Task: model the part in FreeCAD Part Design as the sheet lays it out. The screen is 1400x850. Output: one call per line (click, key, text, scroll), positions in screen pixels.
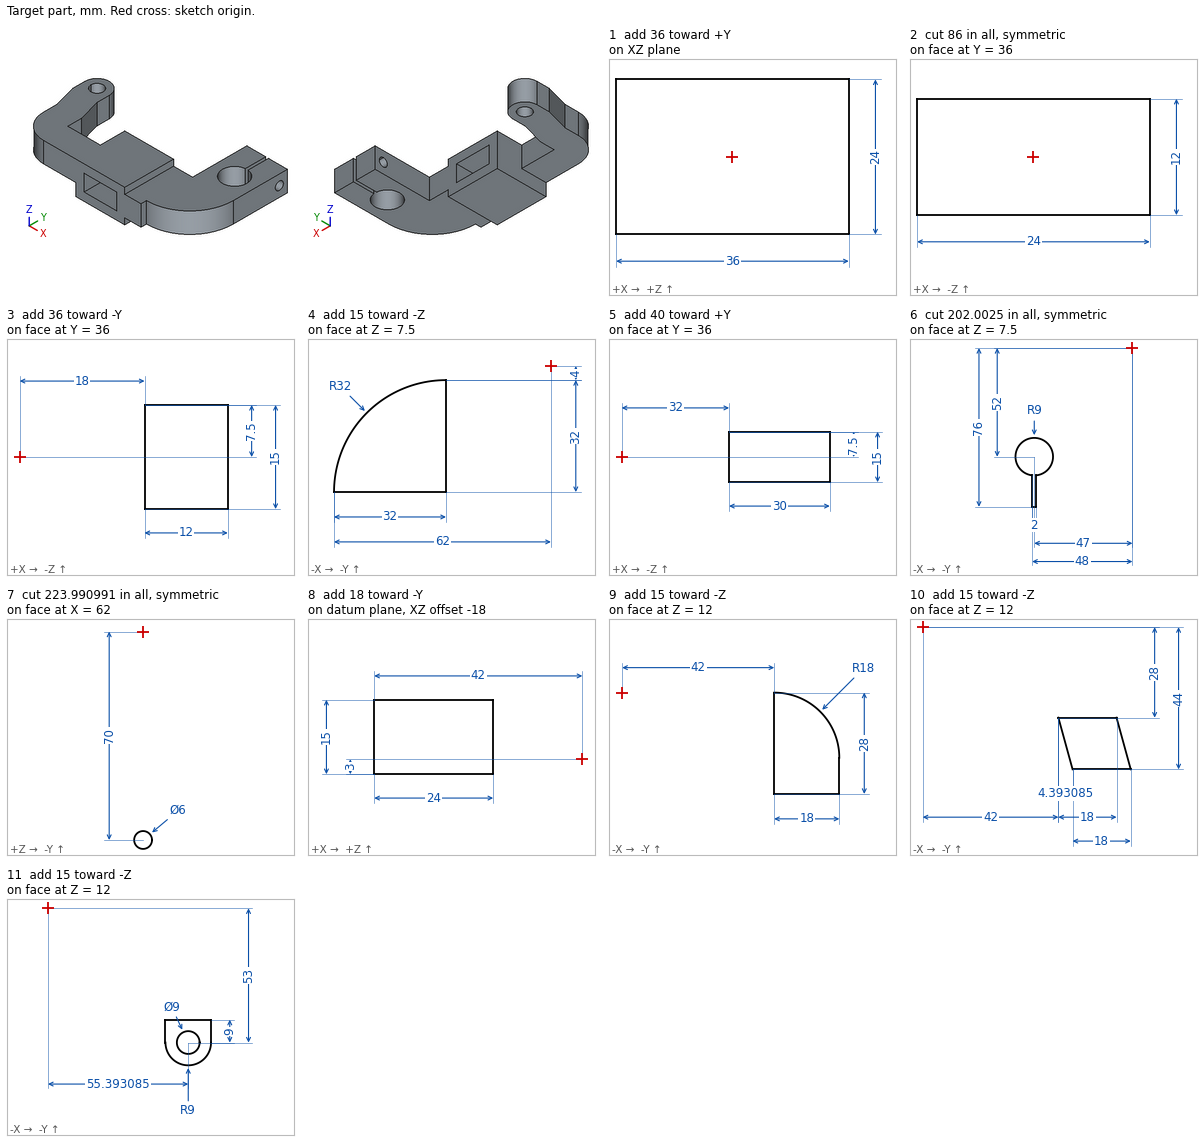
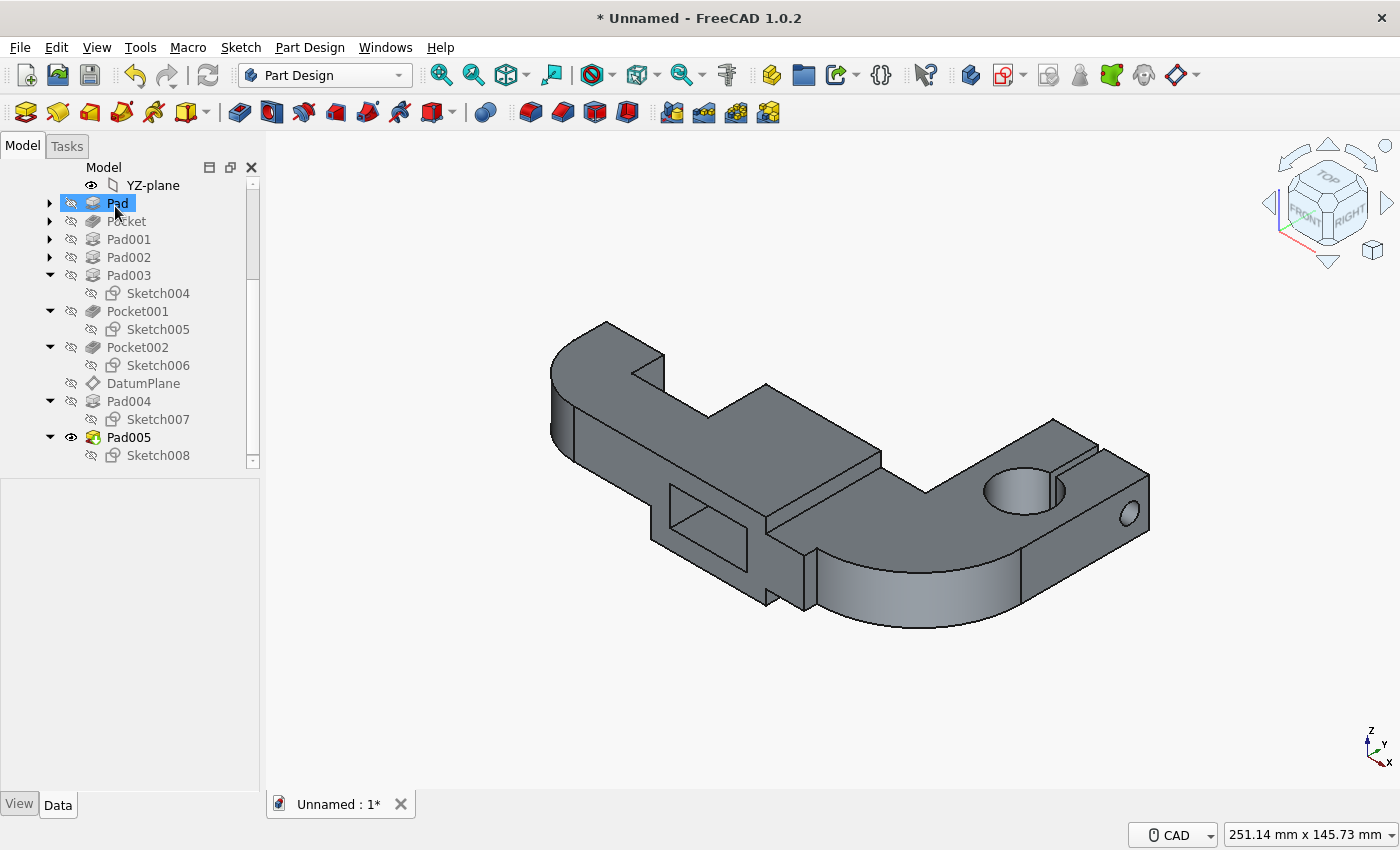
click(770, 452)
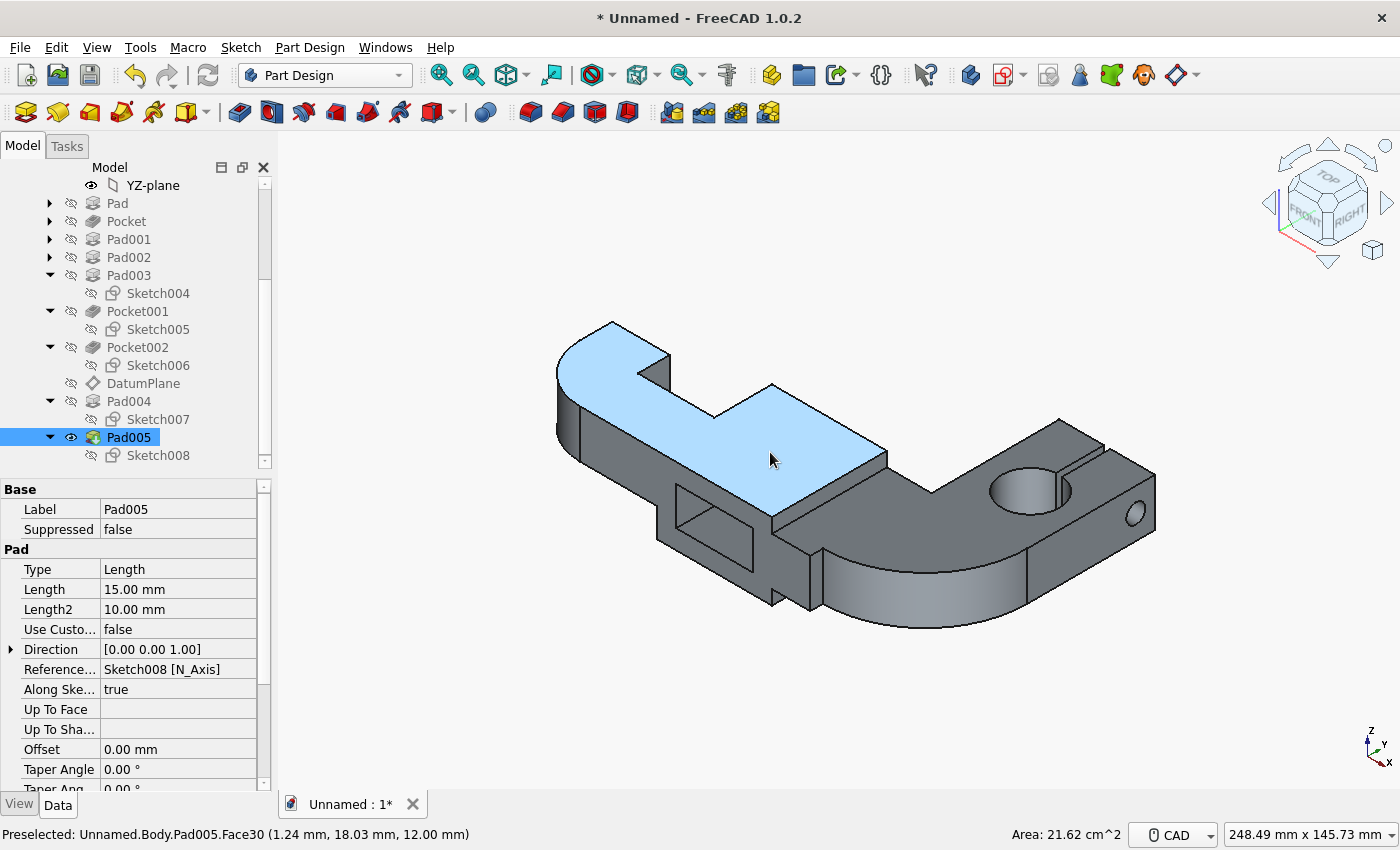
click(1004, 76)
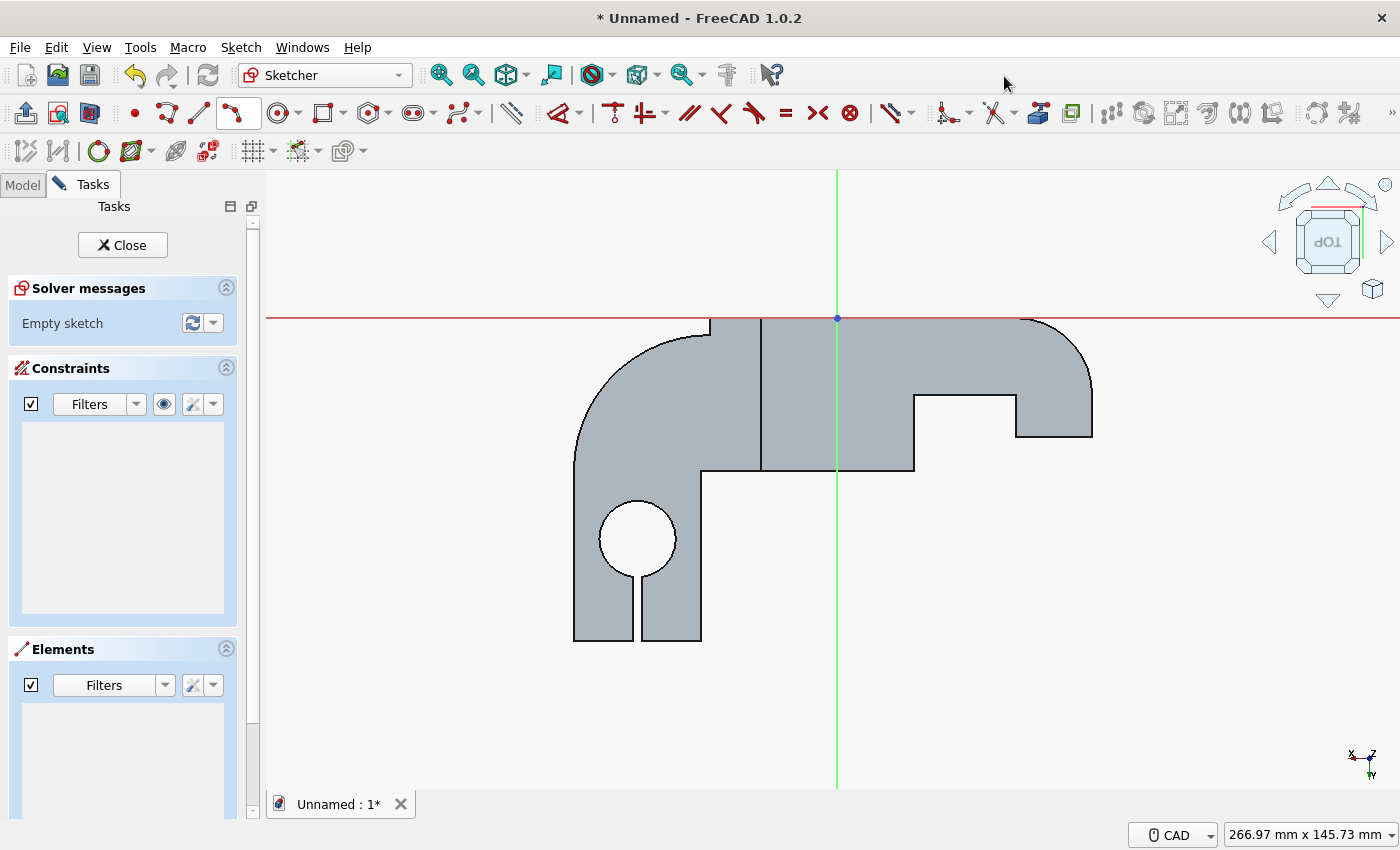
scroll(1122, 469, up, 9)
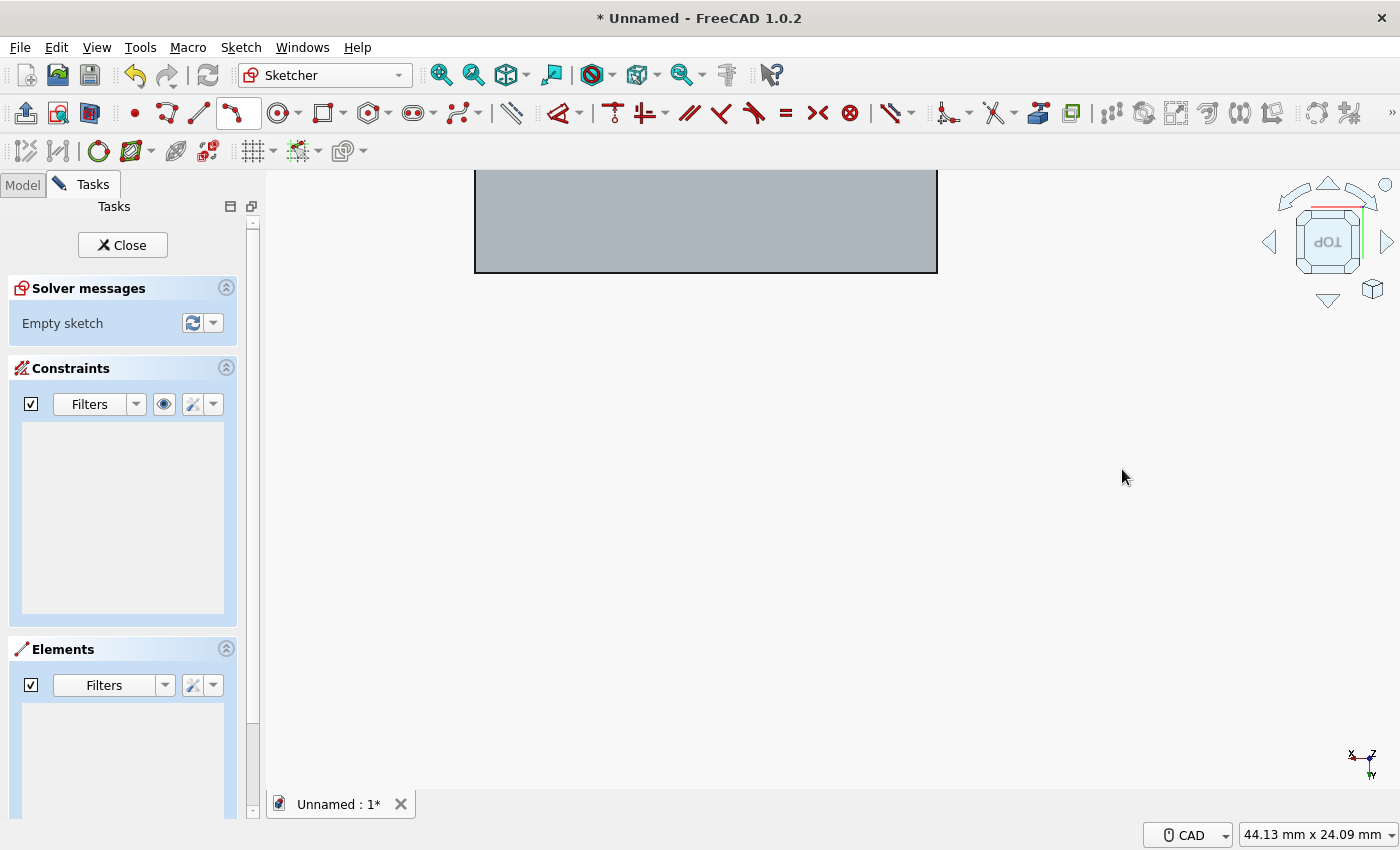
key(g)
key(m)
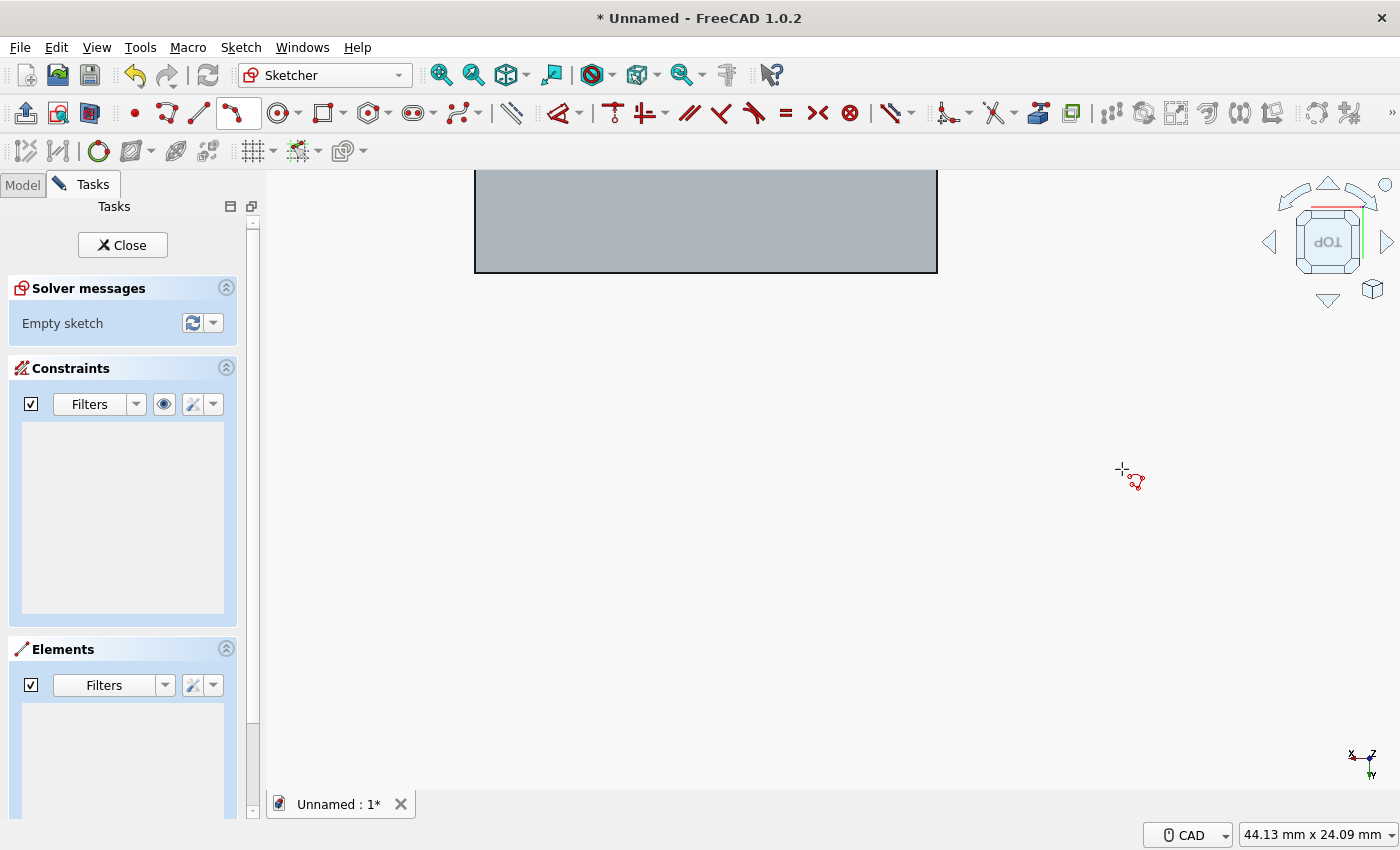
click(475, 273)
click(588, 684)
click(1050, 684)
click(937, 273)
click(475, 274)
key(Escape)
key(Escape)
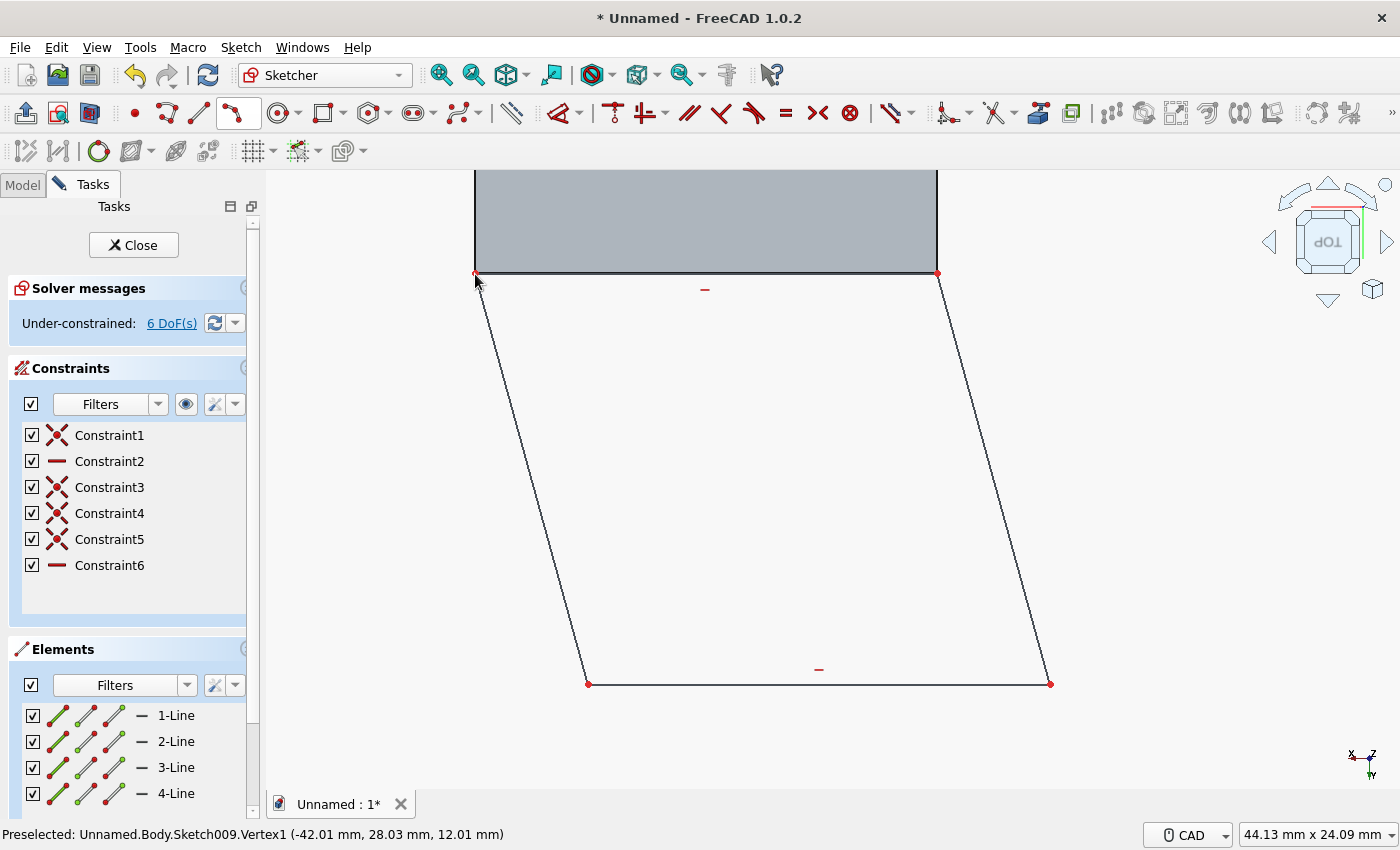
click(558, 114)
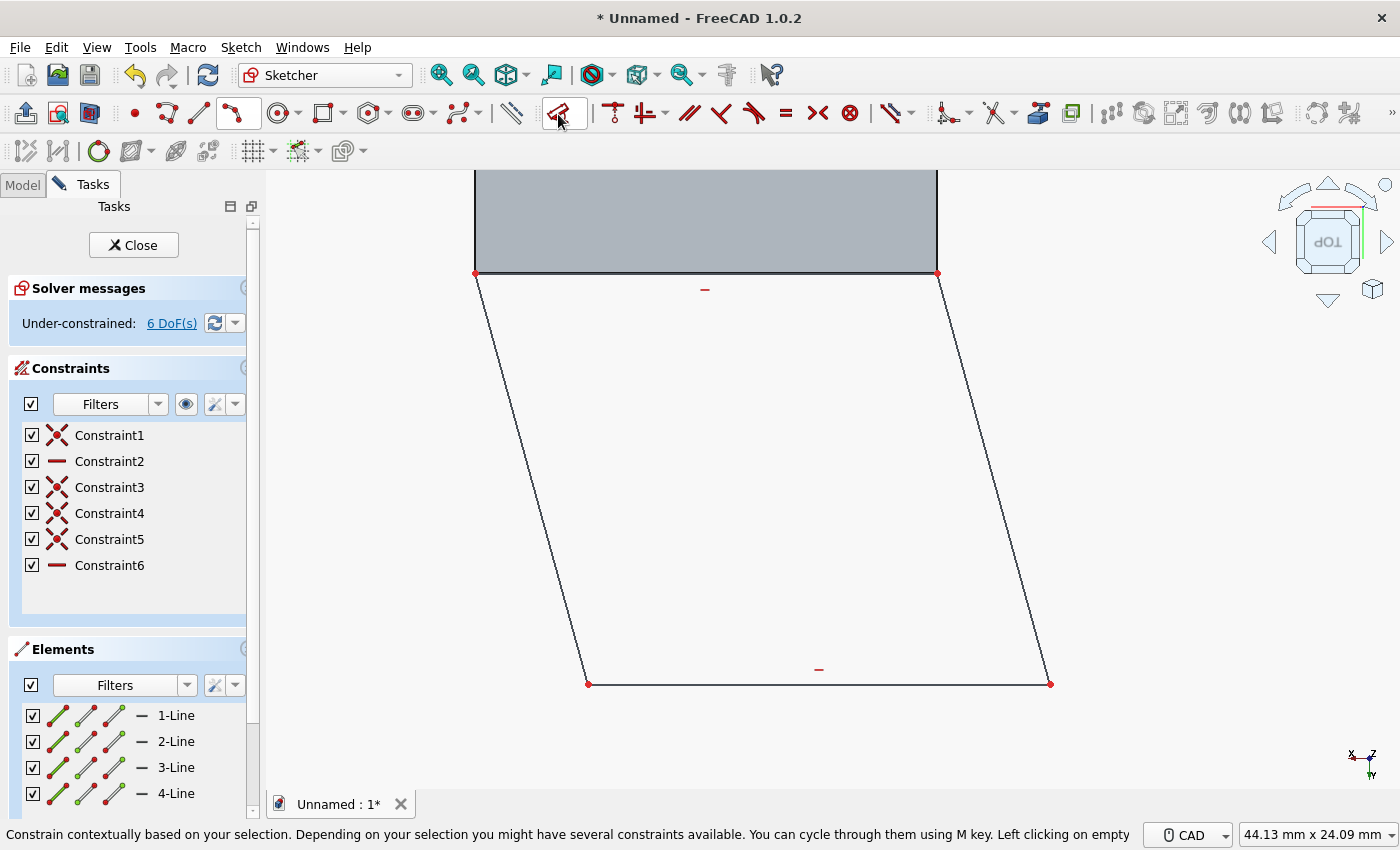
click(727, 685)
click(819, 719)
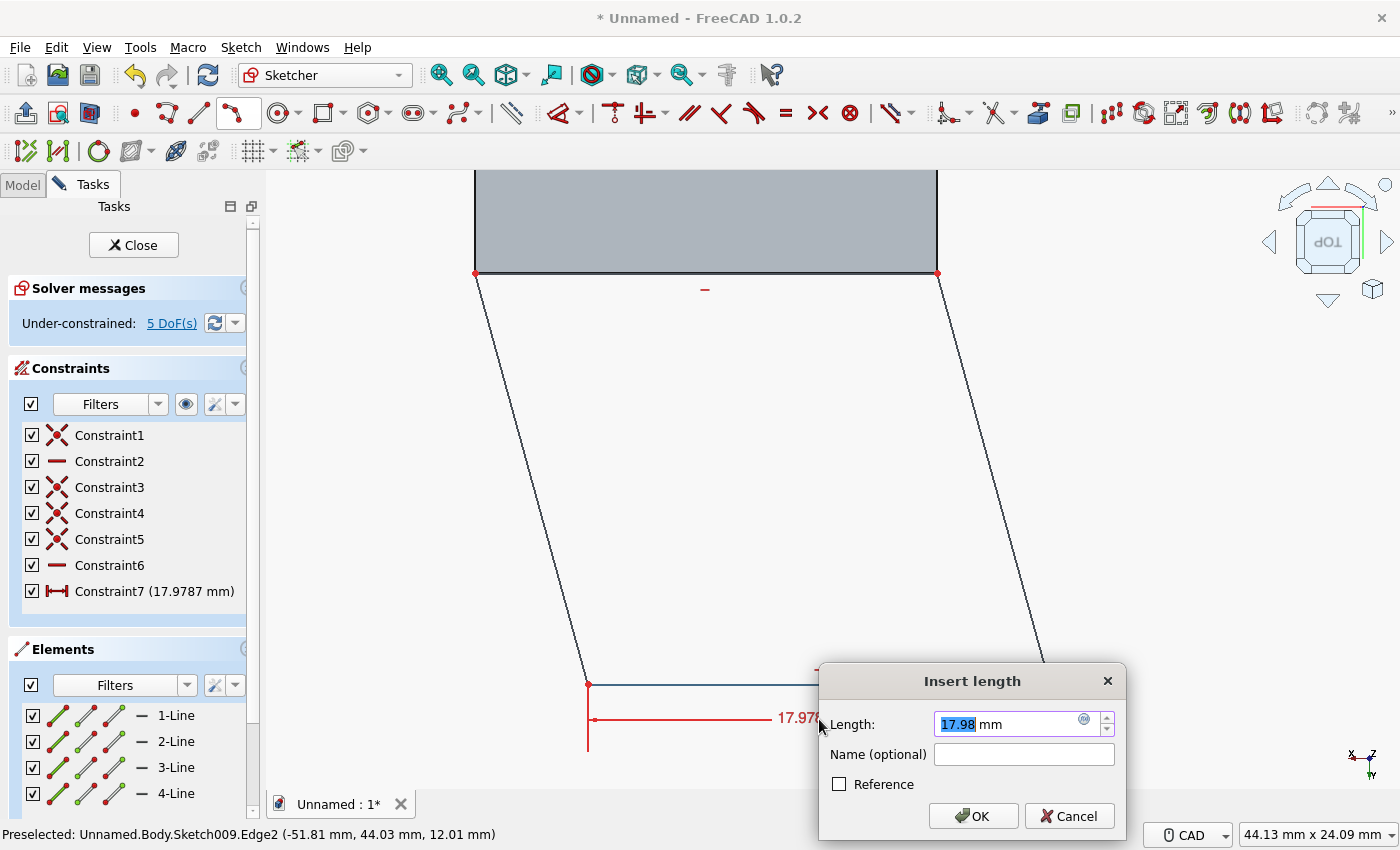
text(18)
key(Return)